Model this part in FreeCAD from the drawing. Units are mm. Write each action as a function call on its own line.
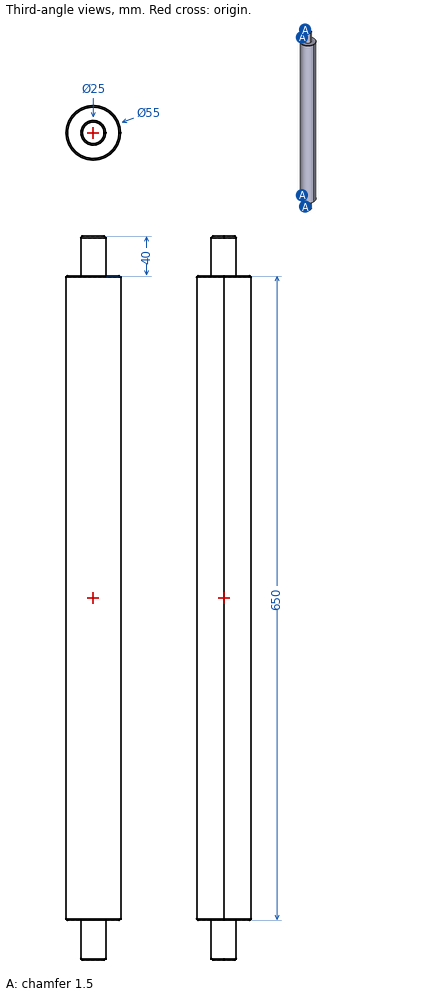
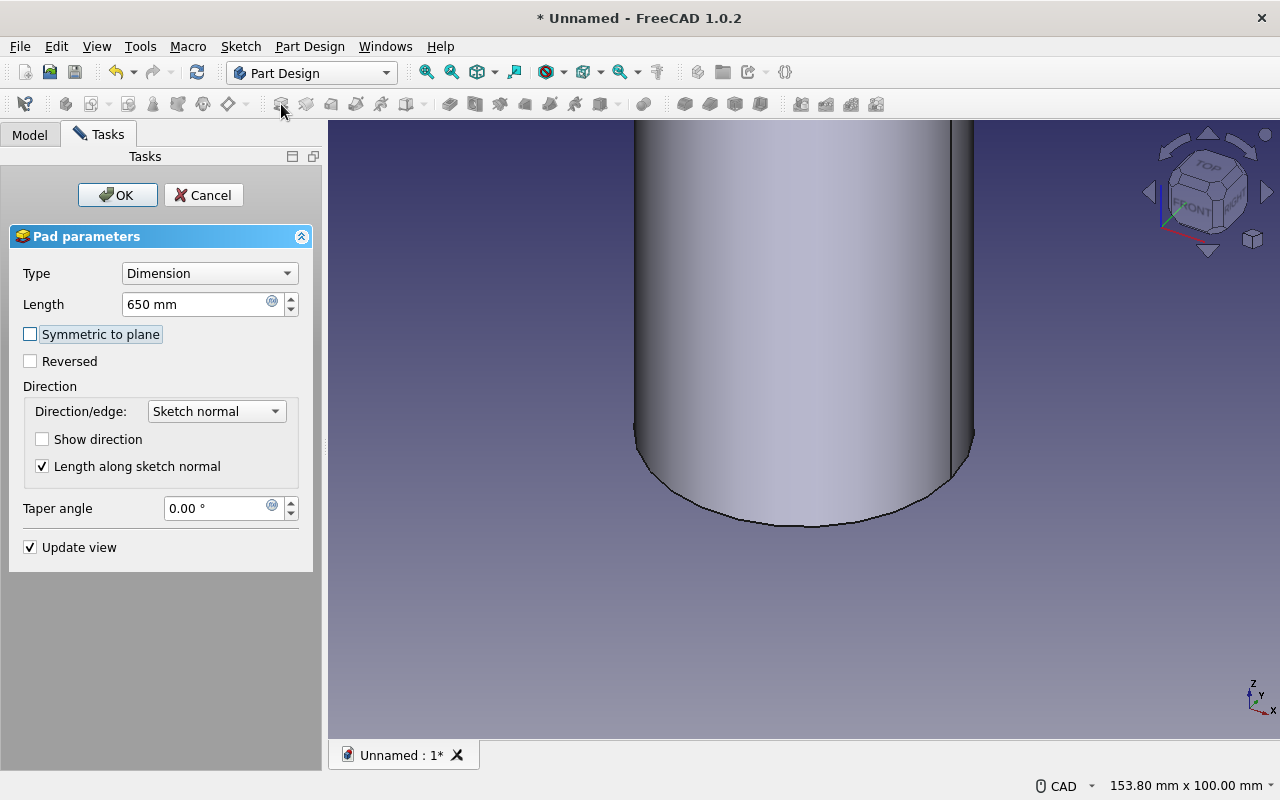
click(31, 334)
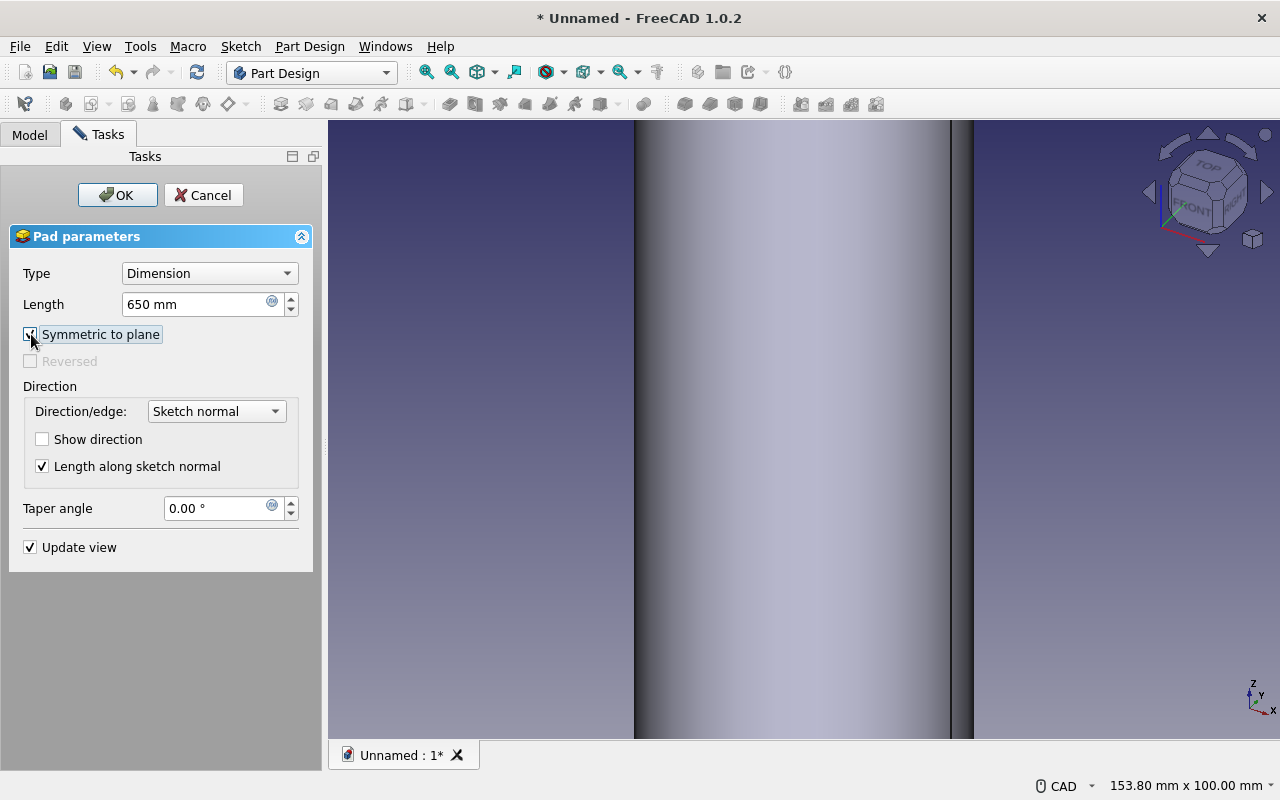
click(118, 195)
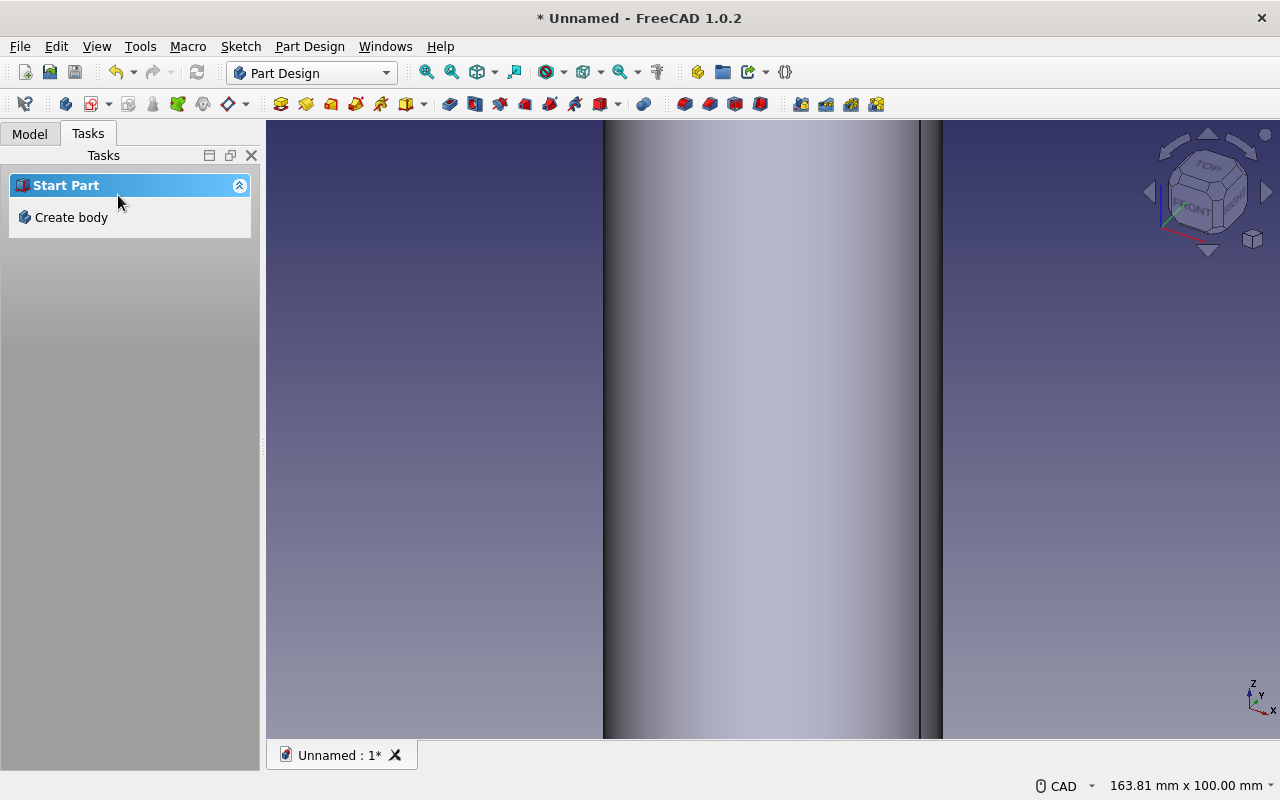
key(v)
key(f)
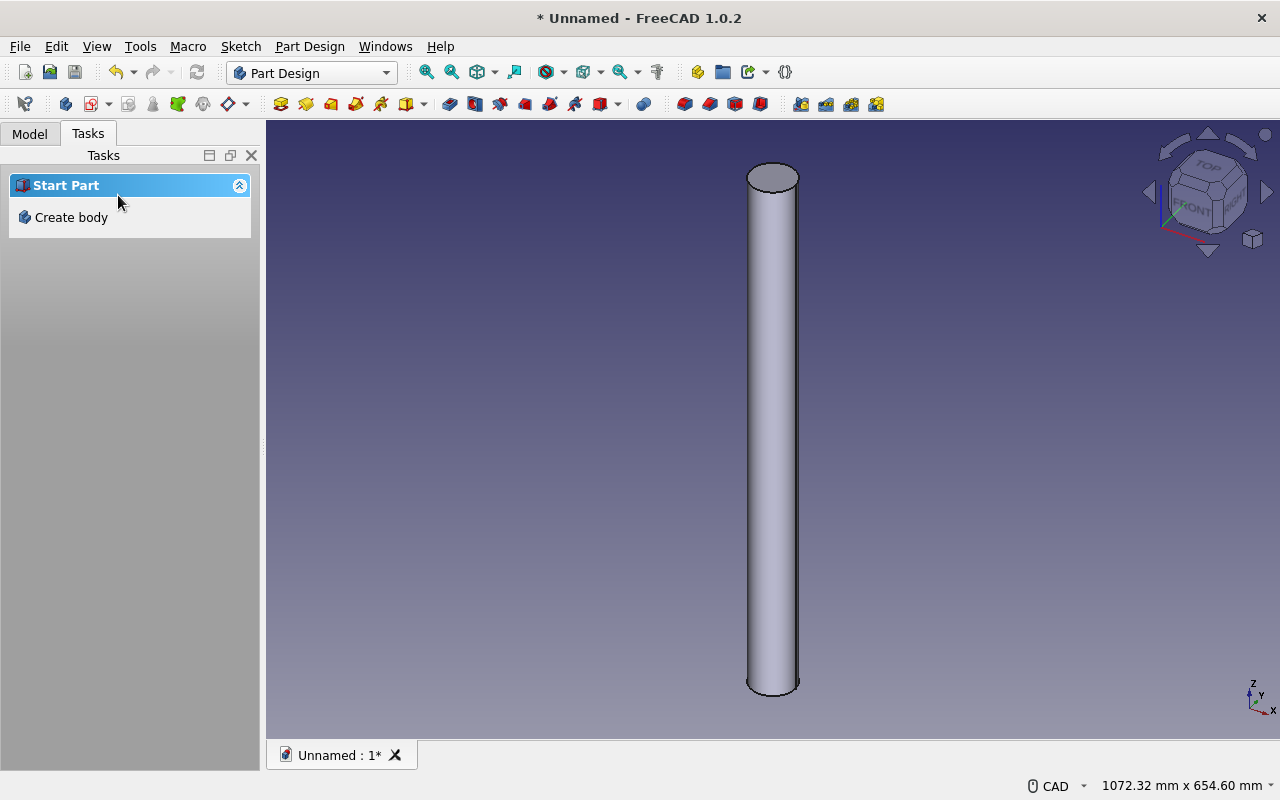
click(773, 177)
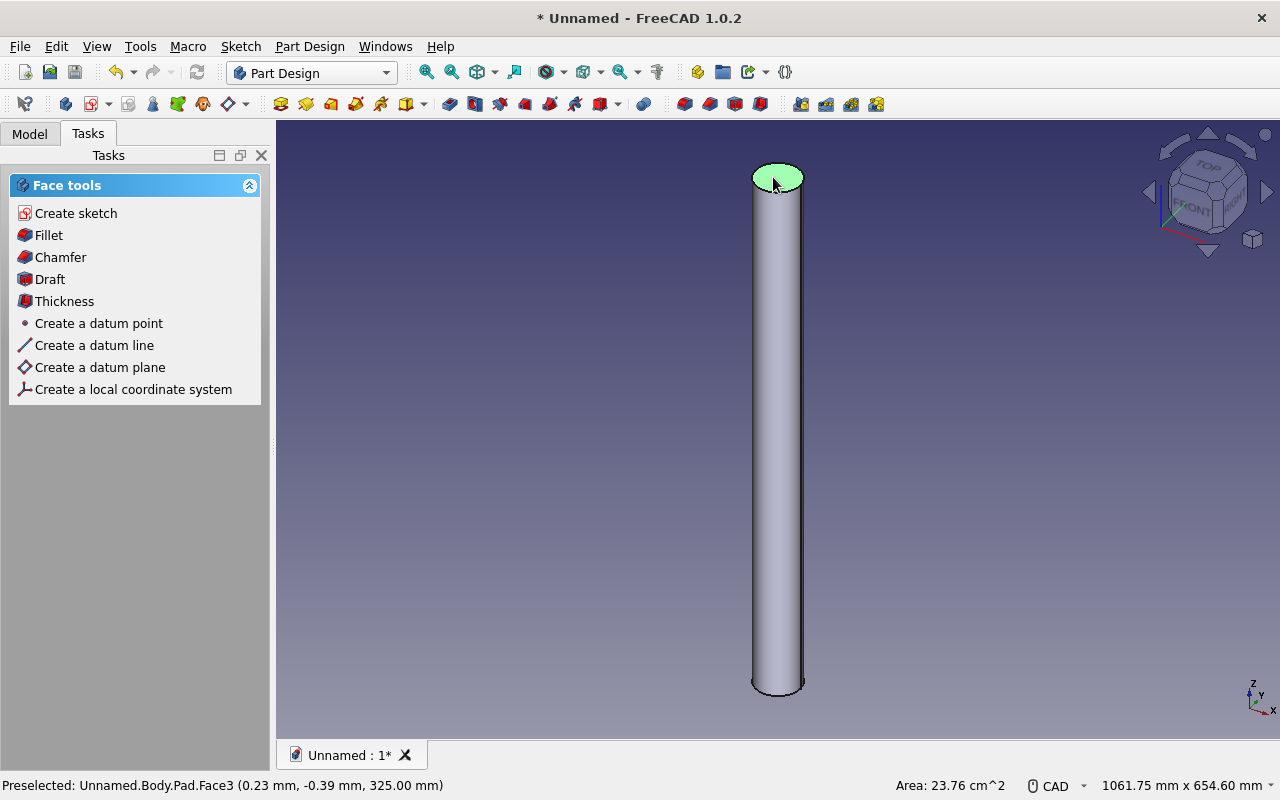
click(90, 104)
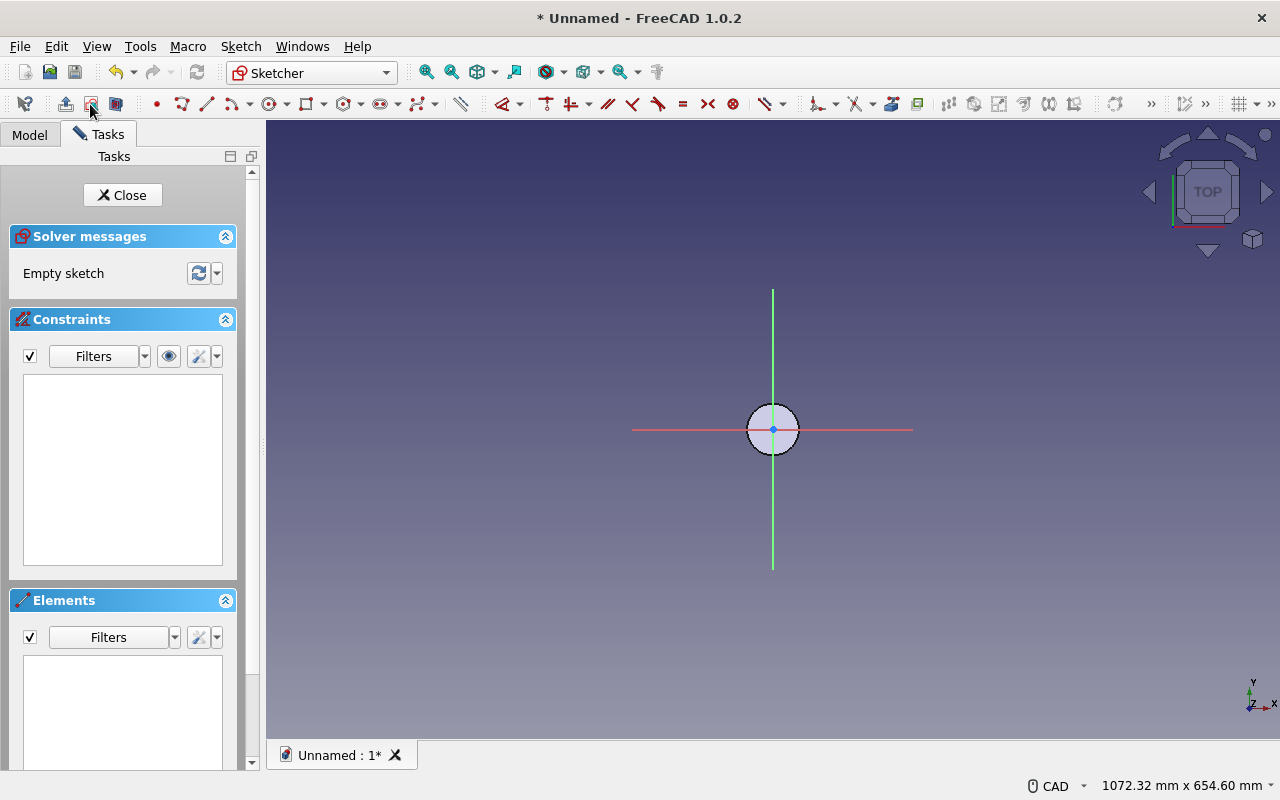
scroll(777, 430, up, 14)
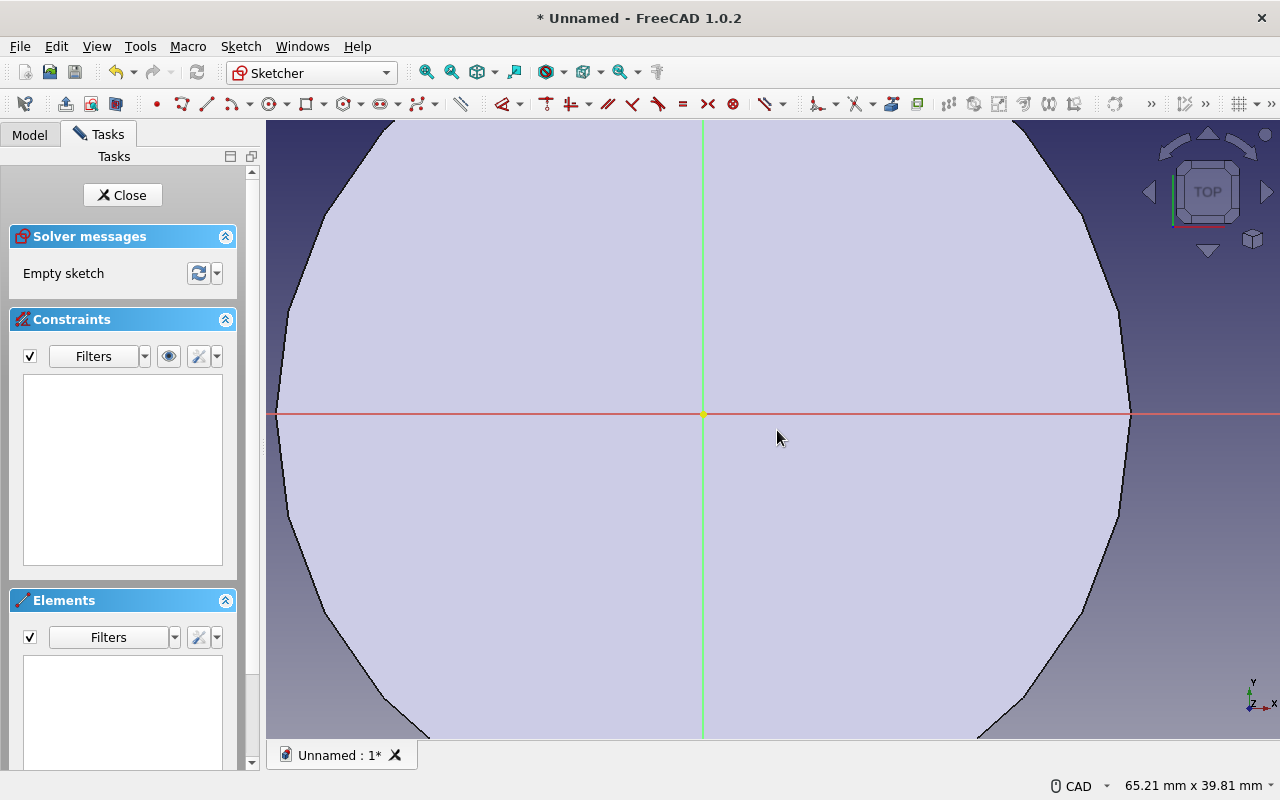
click(268, 104)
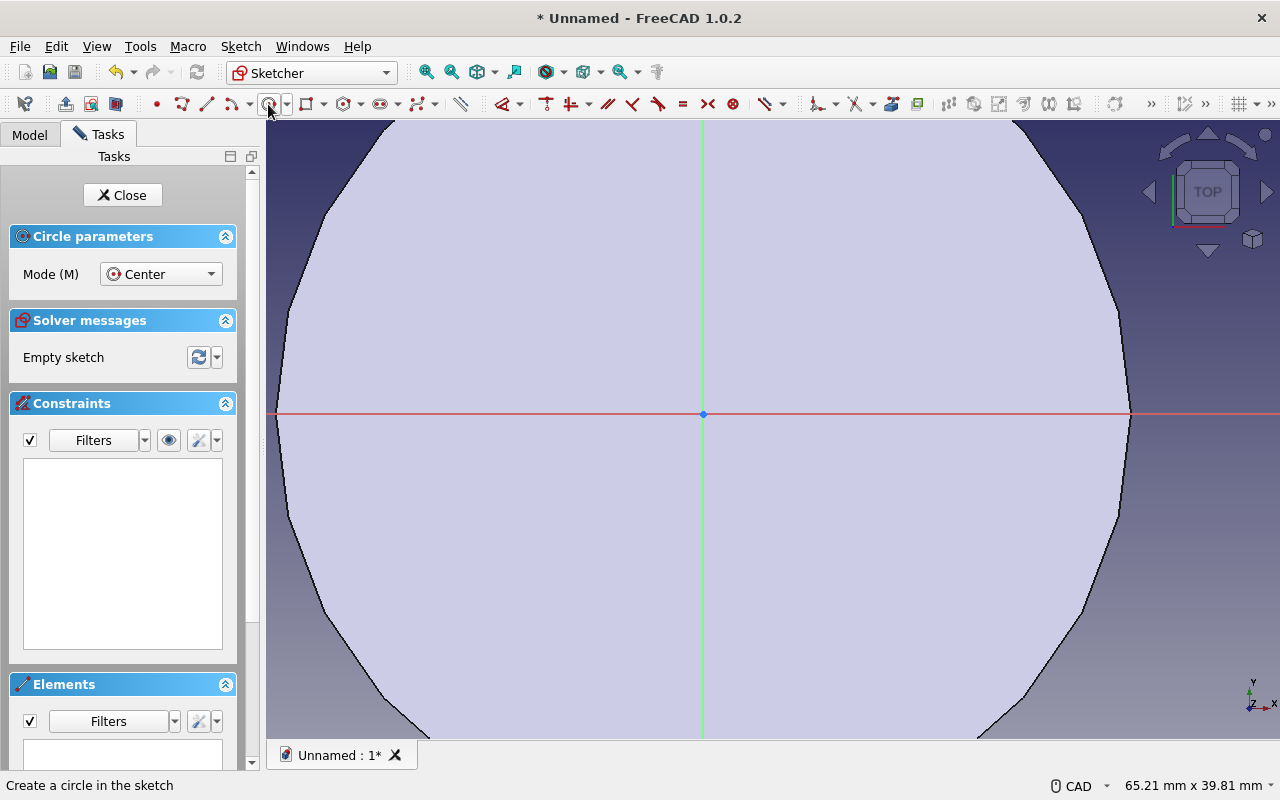
click(703, 414)
move(841, 277)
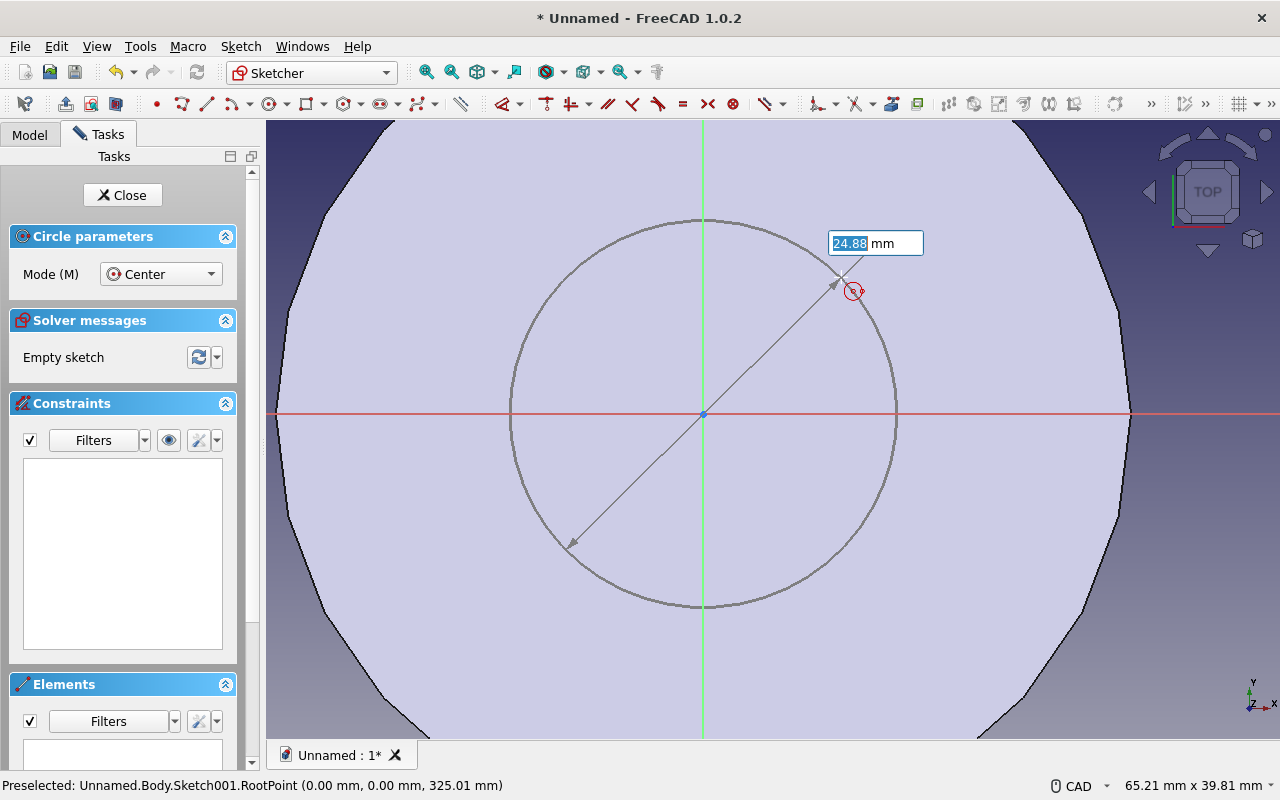
text(25)
key(Return)
key(Escape)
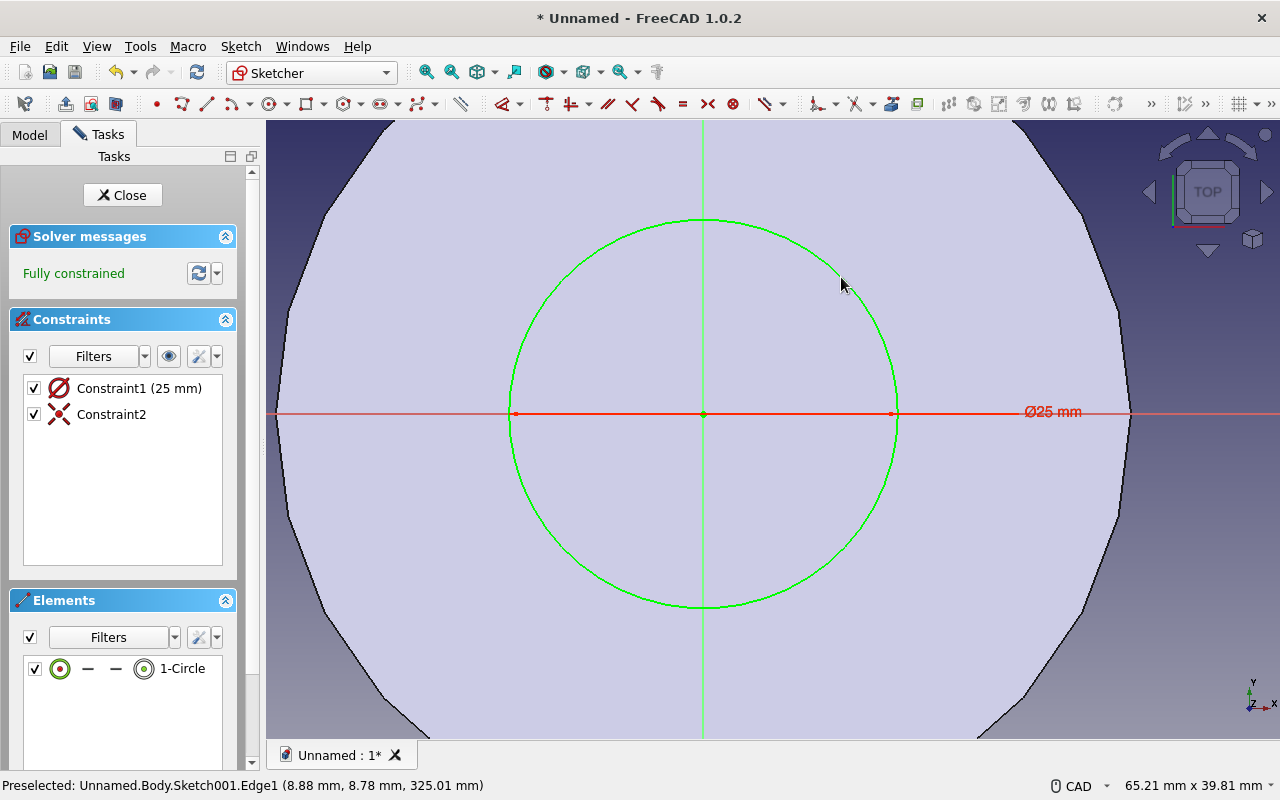
click(123, 195)